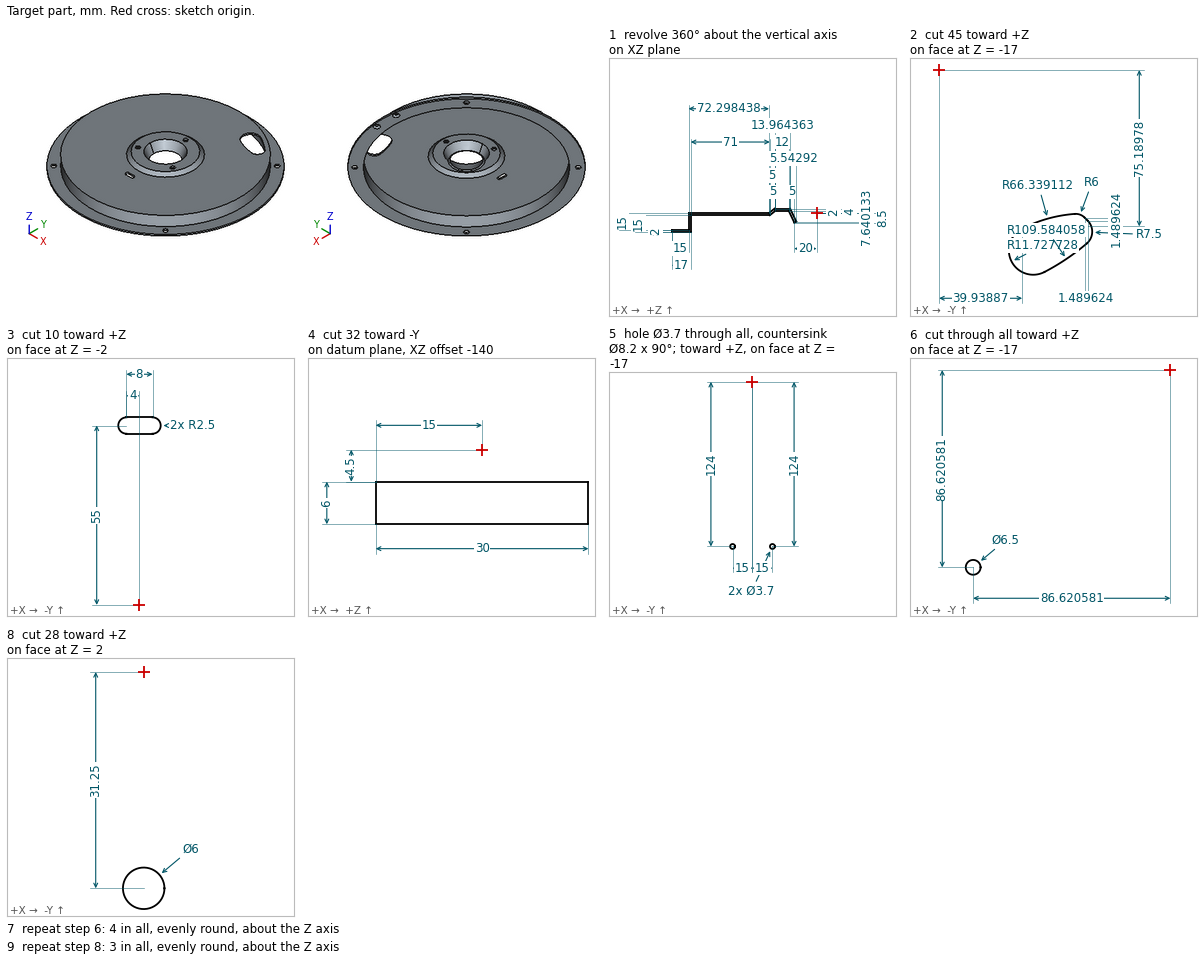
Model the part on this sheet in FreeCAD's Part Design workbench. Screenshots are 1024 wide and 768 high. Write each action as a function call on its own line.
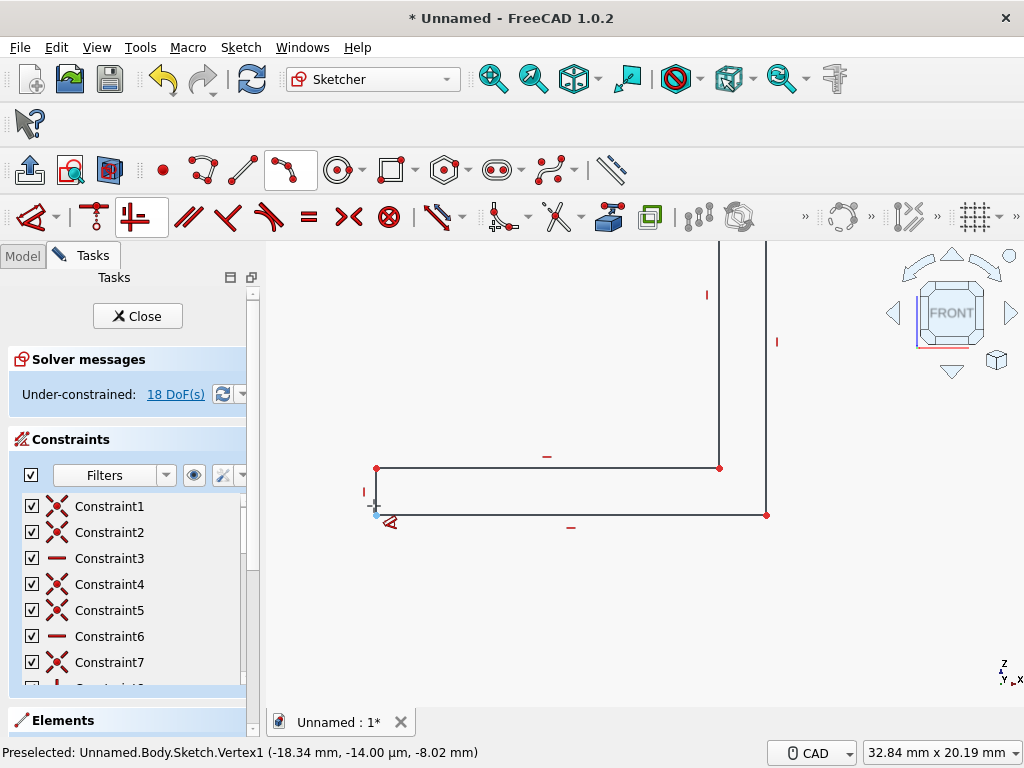
click(376, 501)
click(342, 492)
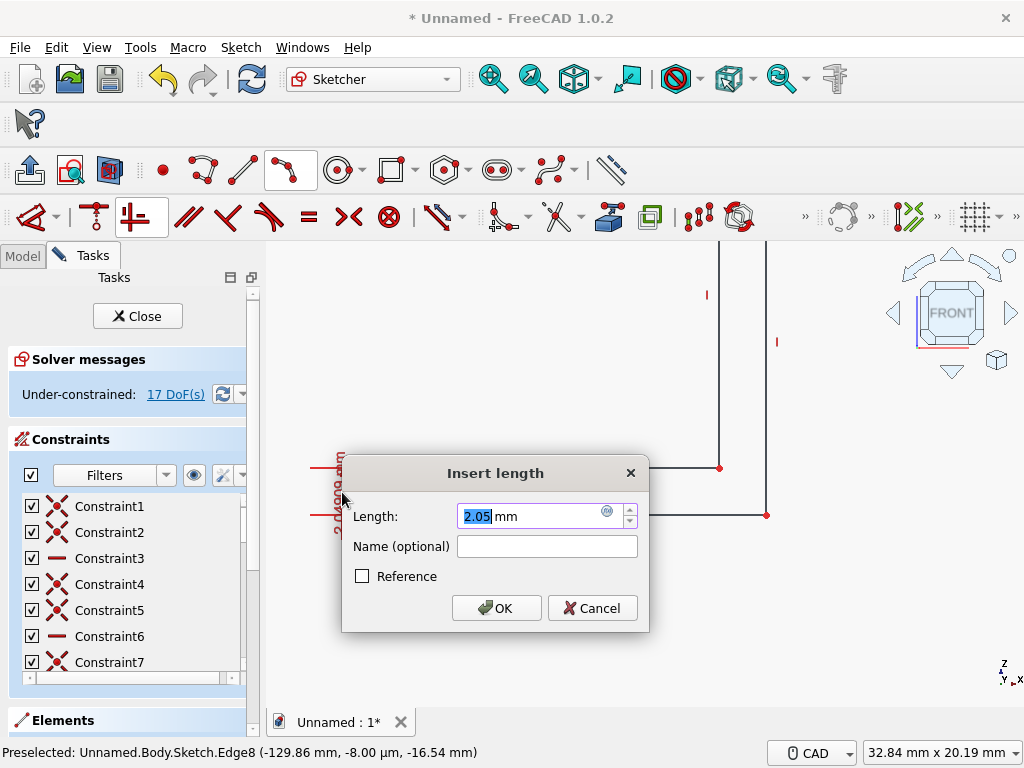
text(2)
key(Return)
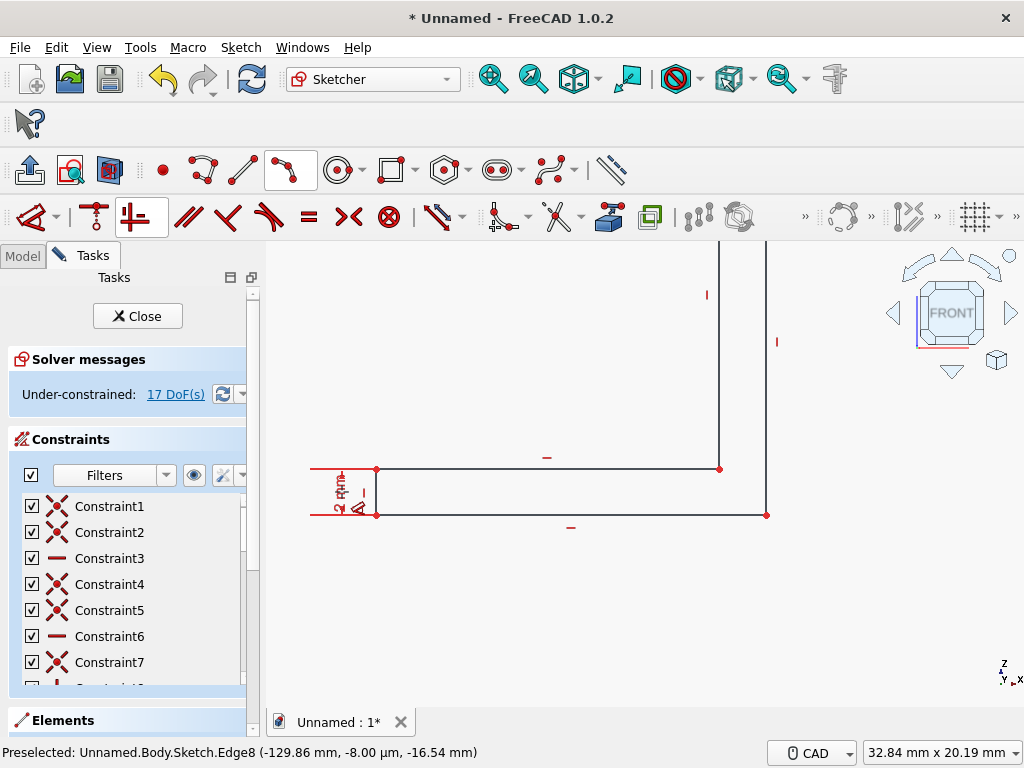
scroll(374, 506, down, 10)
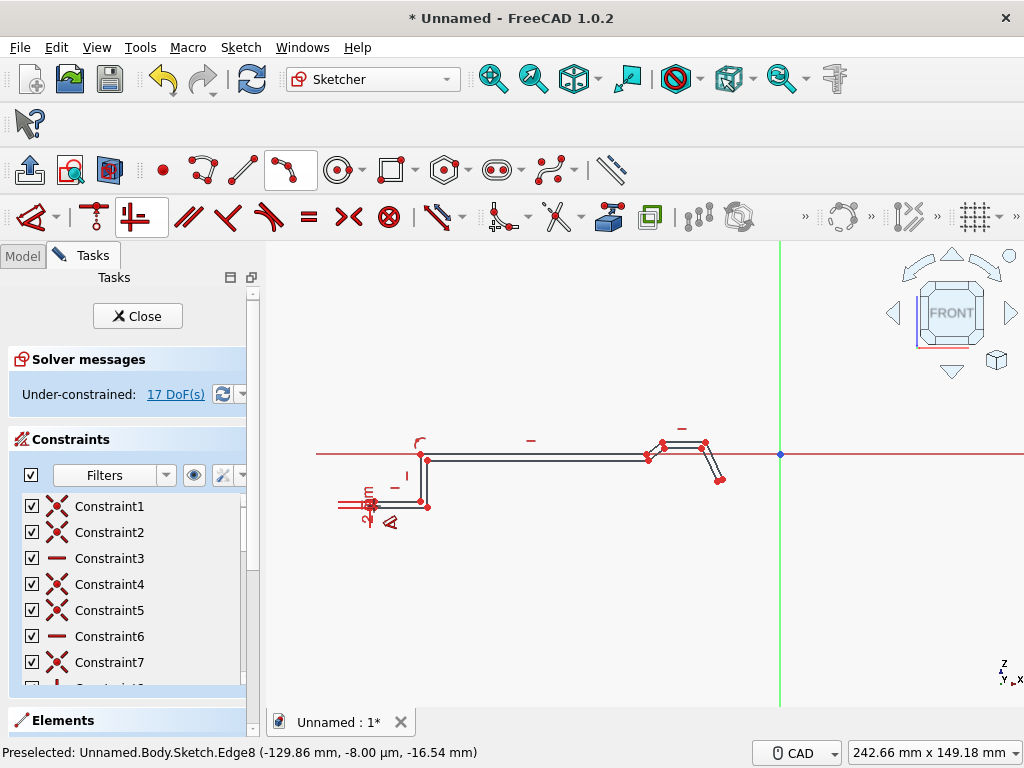
scroll(691, 448, up, 5)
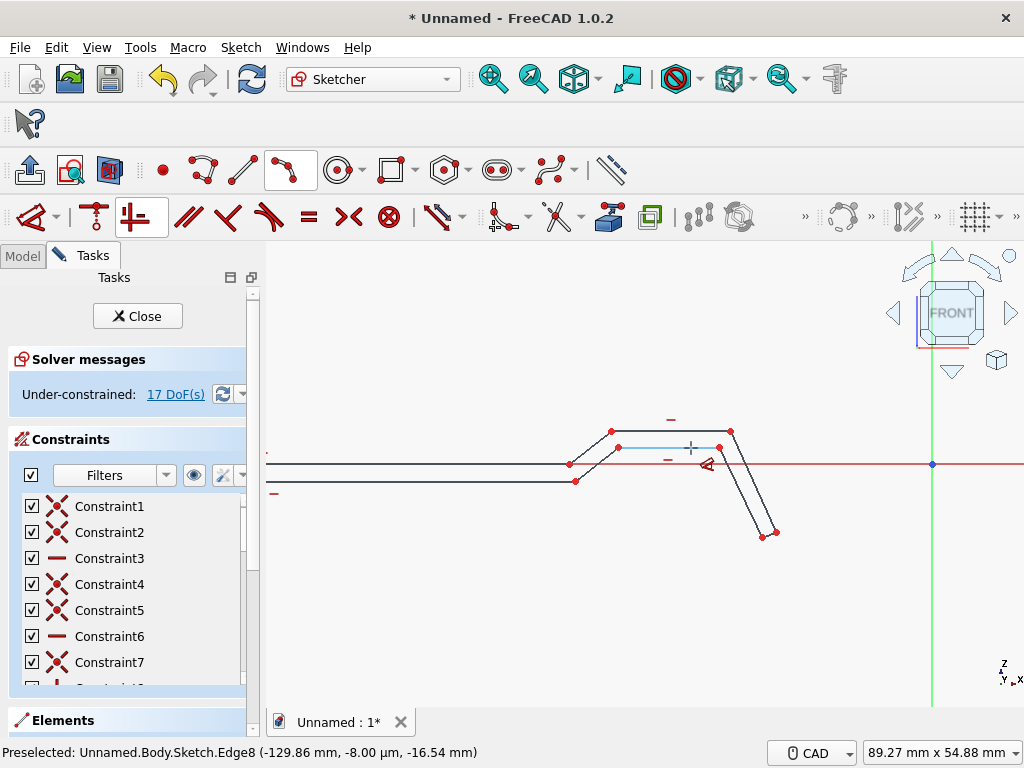
click(689, 448)
click(669, 414)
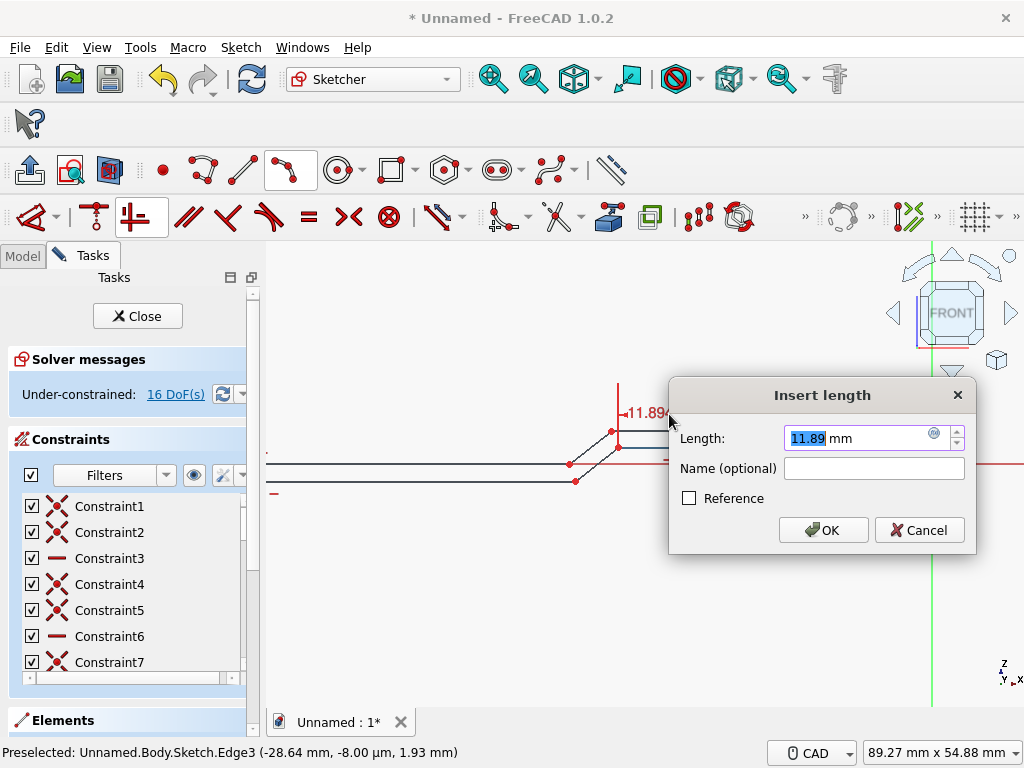
text(12)
key(Return)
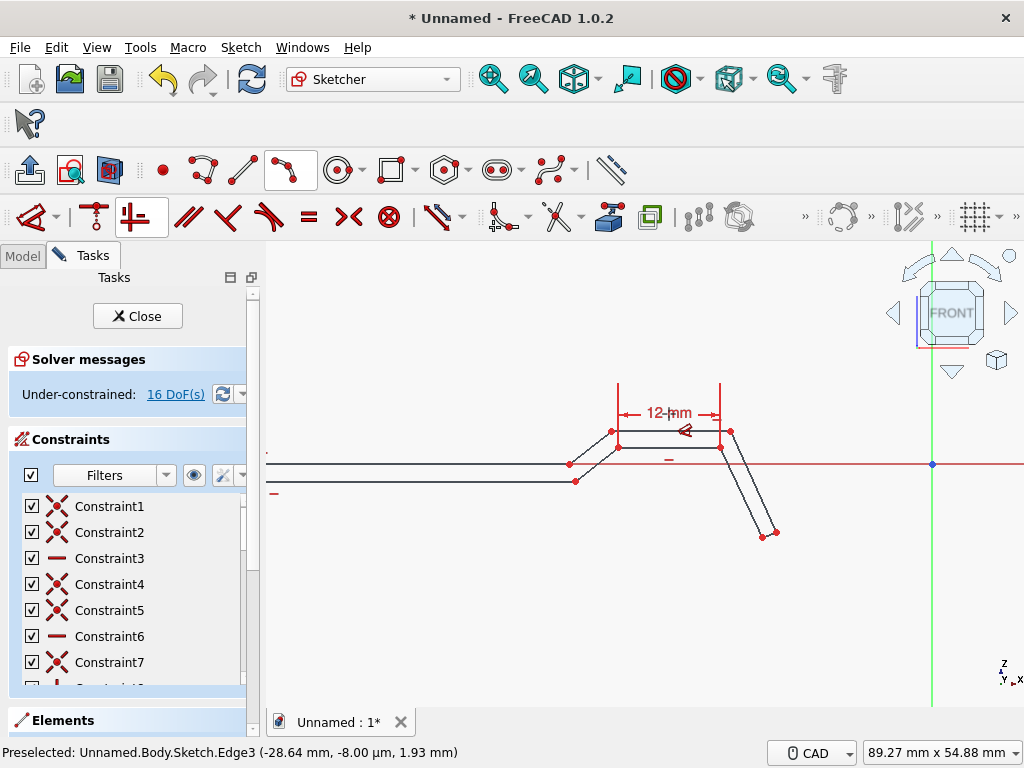
click(395, 482)
click(435, 448)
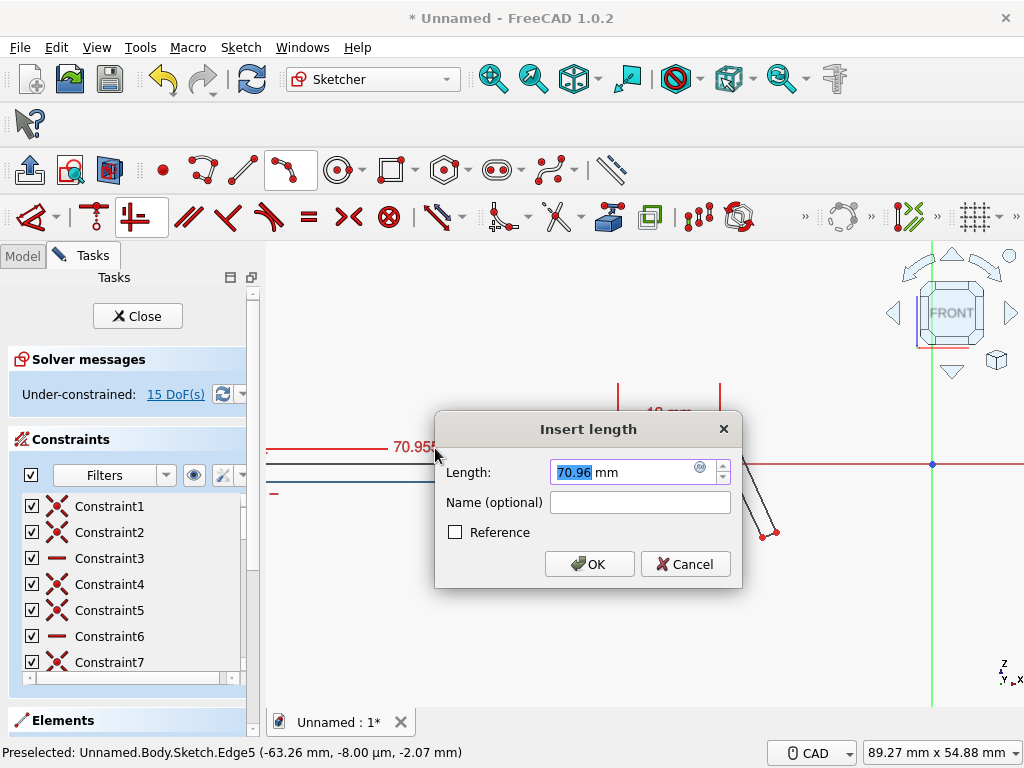
text(71)
key(Return)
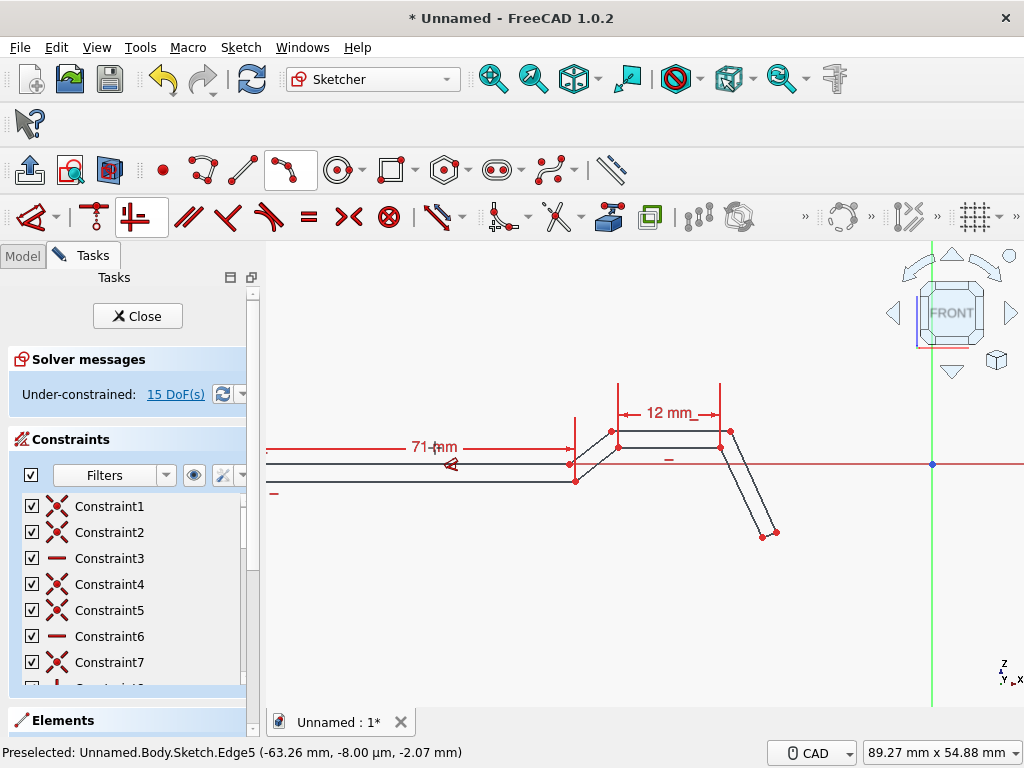
scroll(691, 448, down, 5)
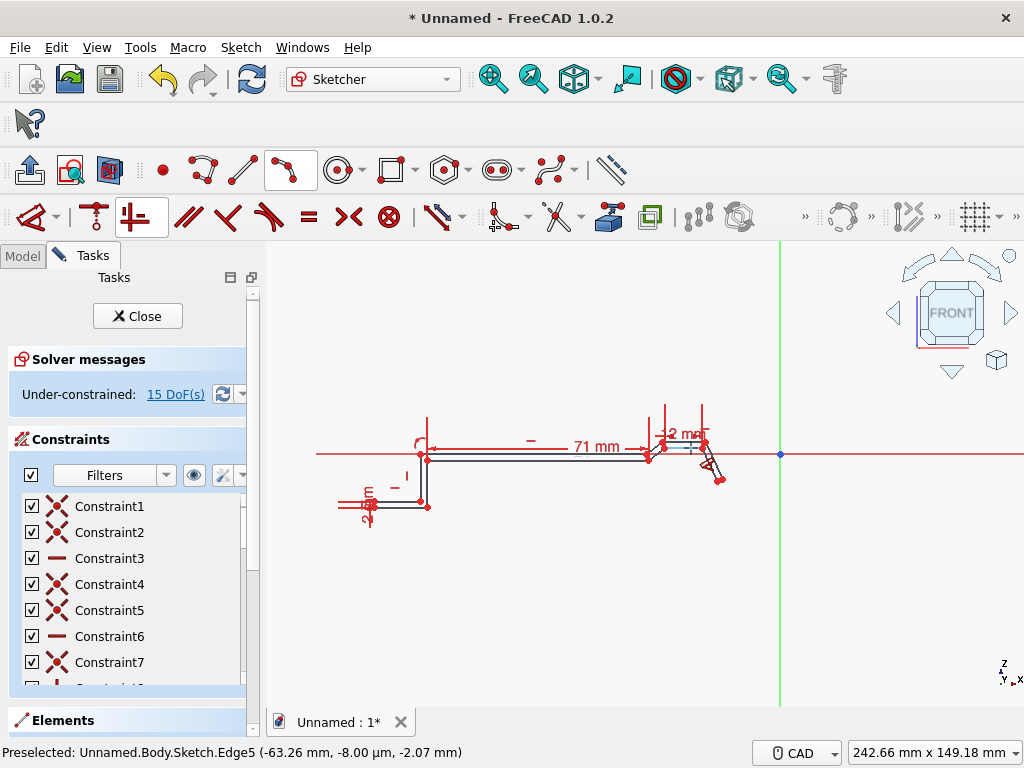
scroll(427, 475, up, 5)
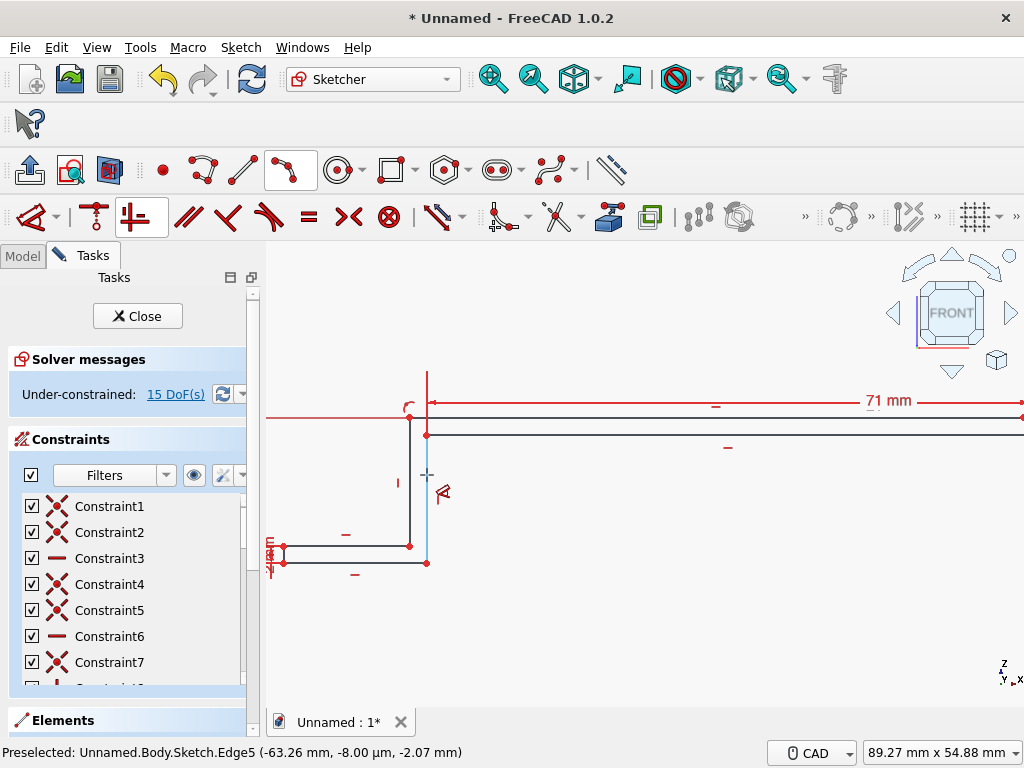
click(427, 474)
click(393, 499)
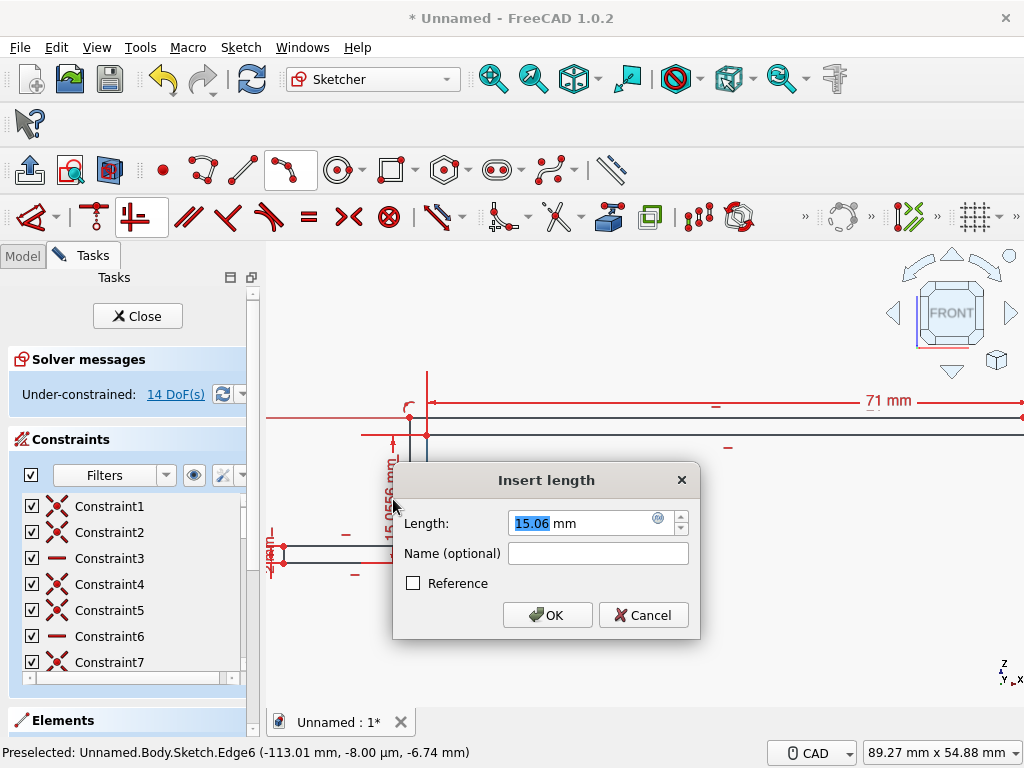
text(15)
key(Return)